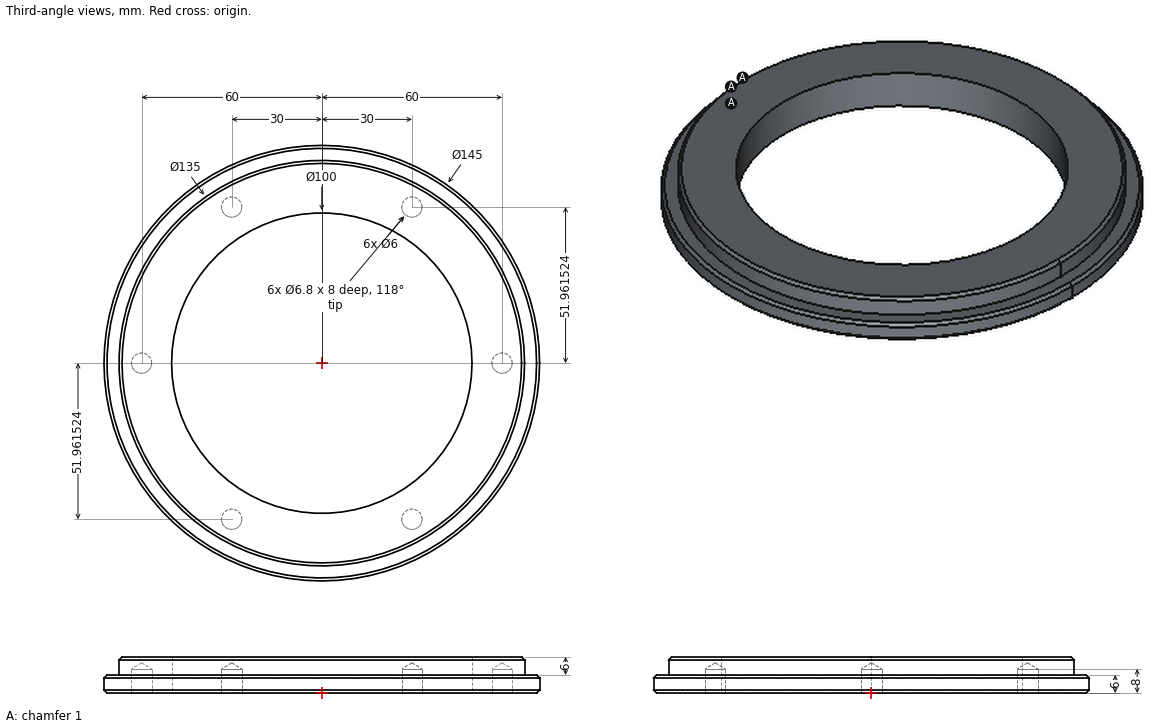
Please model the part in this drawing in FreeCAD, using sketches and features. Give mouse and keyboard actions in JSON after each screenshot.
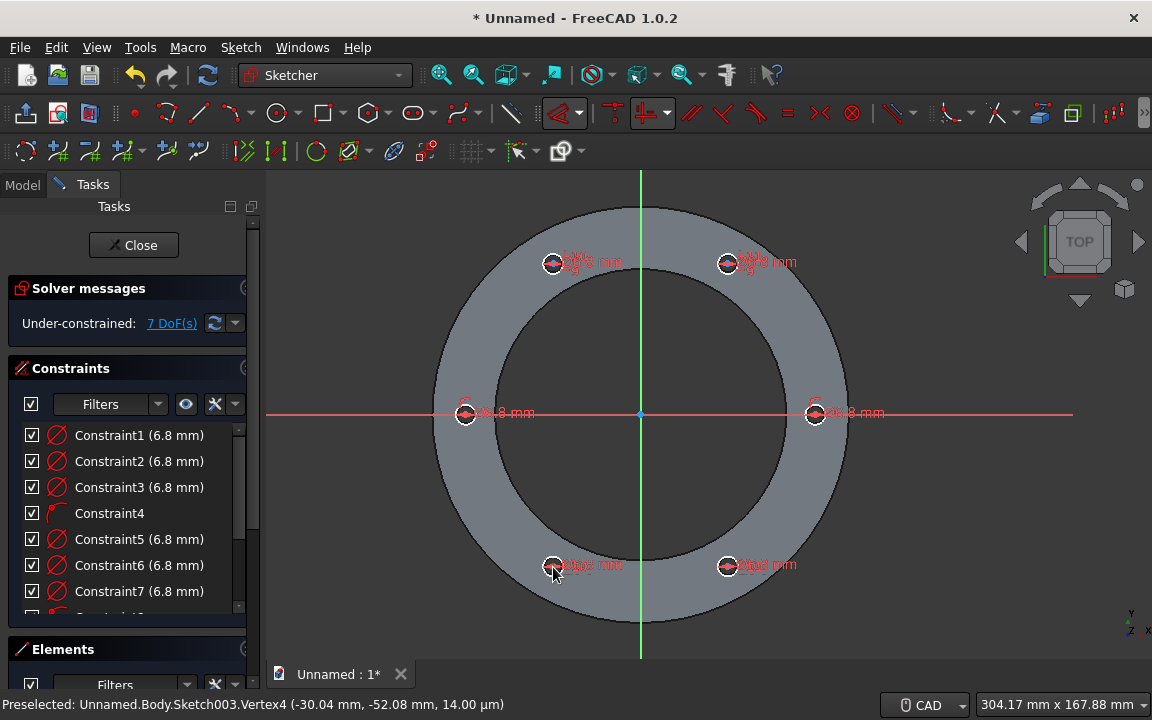
{"action": "left_click", "coordinate": [728, 567]}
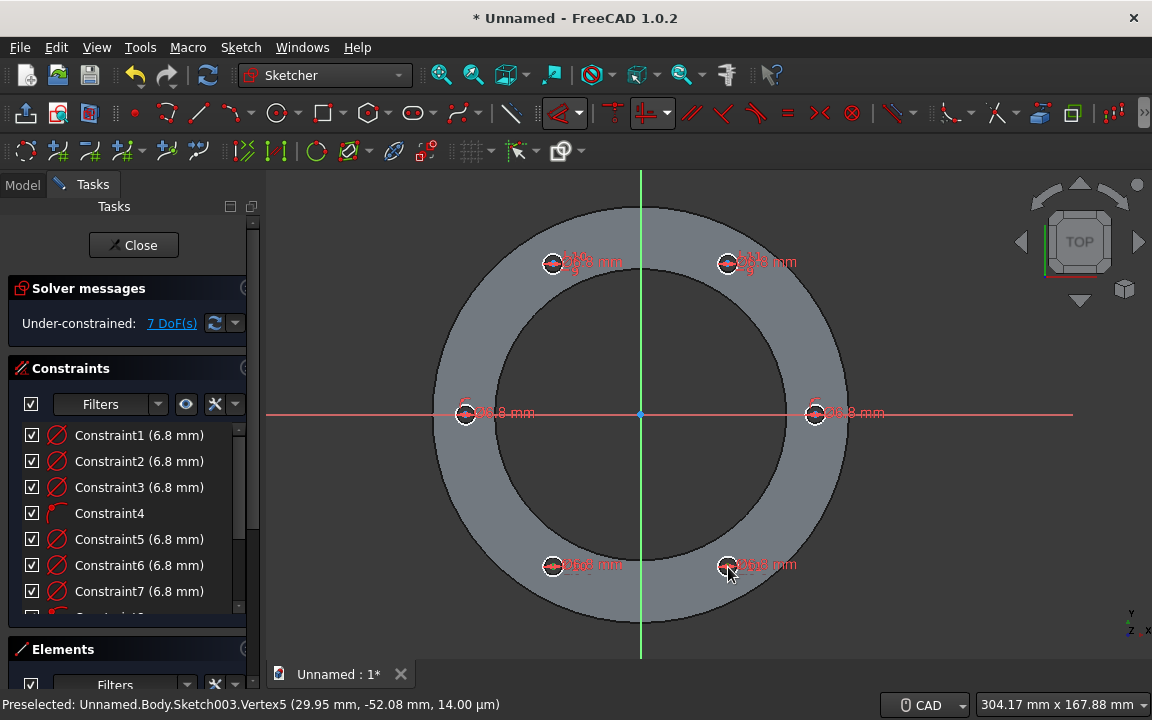
{"action": "left_click", "coordinate": [670, 114]}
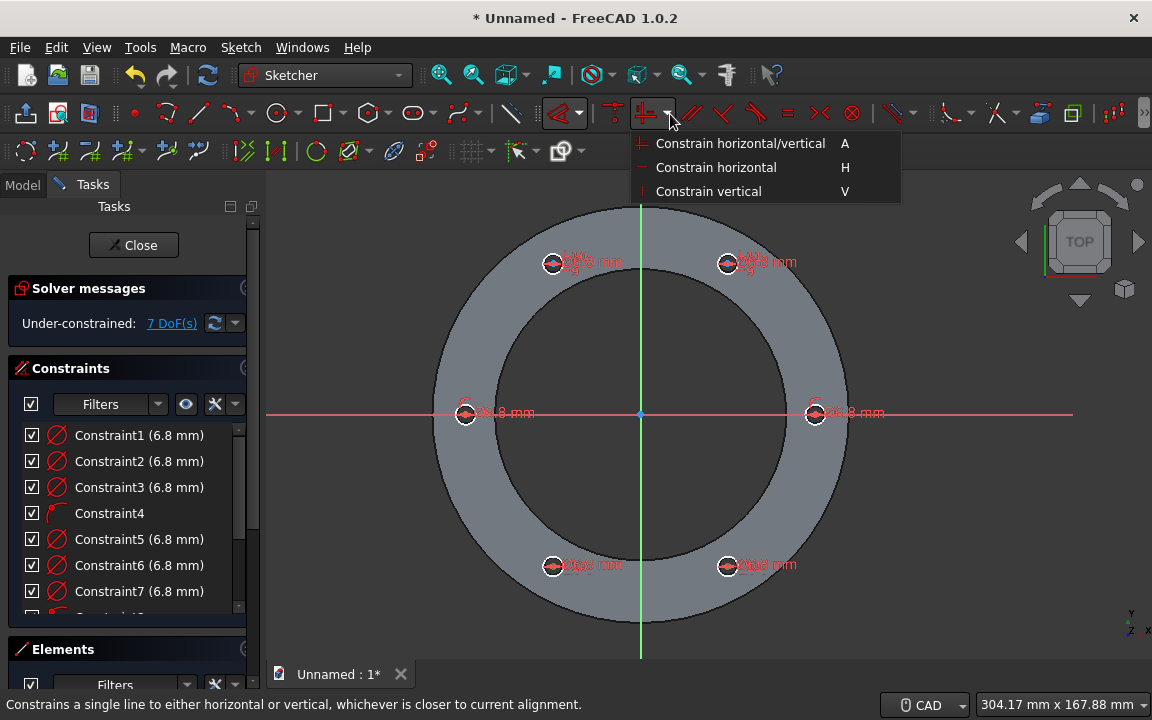
{"action": "left_click", "coordinate": [766, 167]}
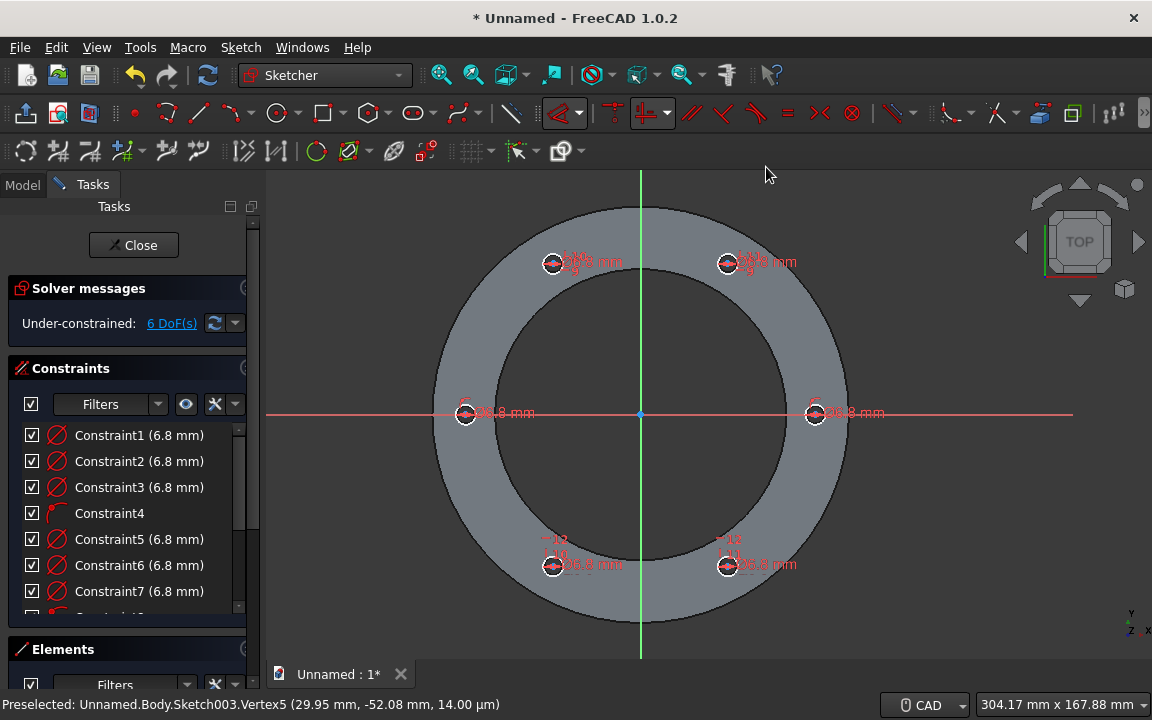
{"action": "left_click", "coordinate": [728, 264]}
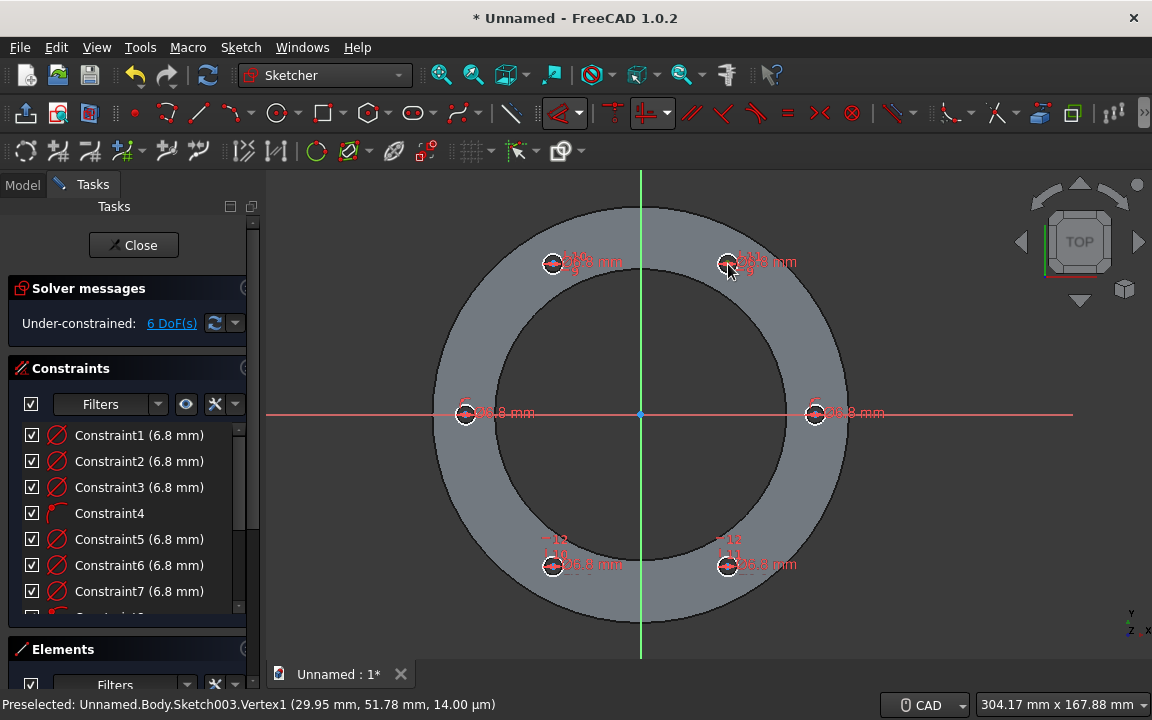
{"action": "key", "text": "l"}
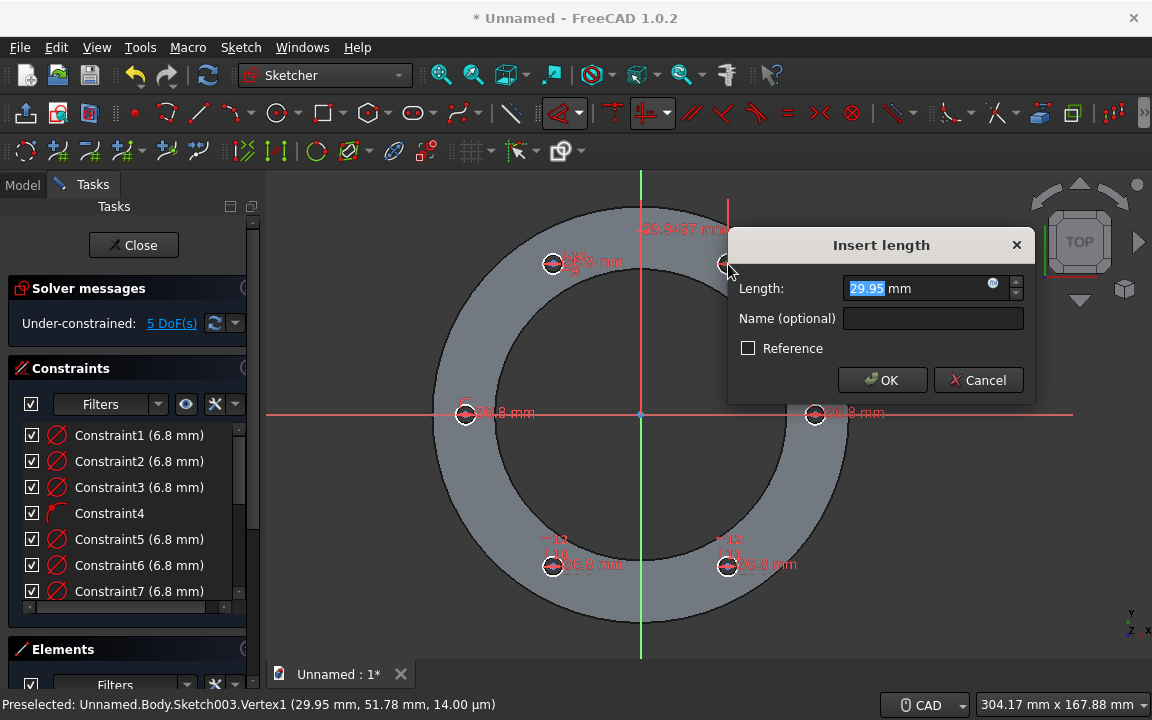
{"action": "type", "text": "30"}
{"action": "key", "text": "Return"}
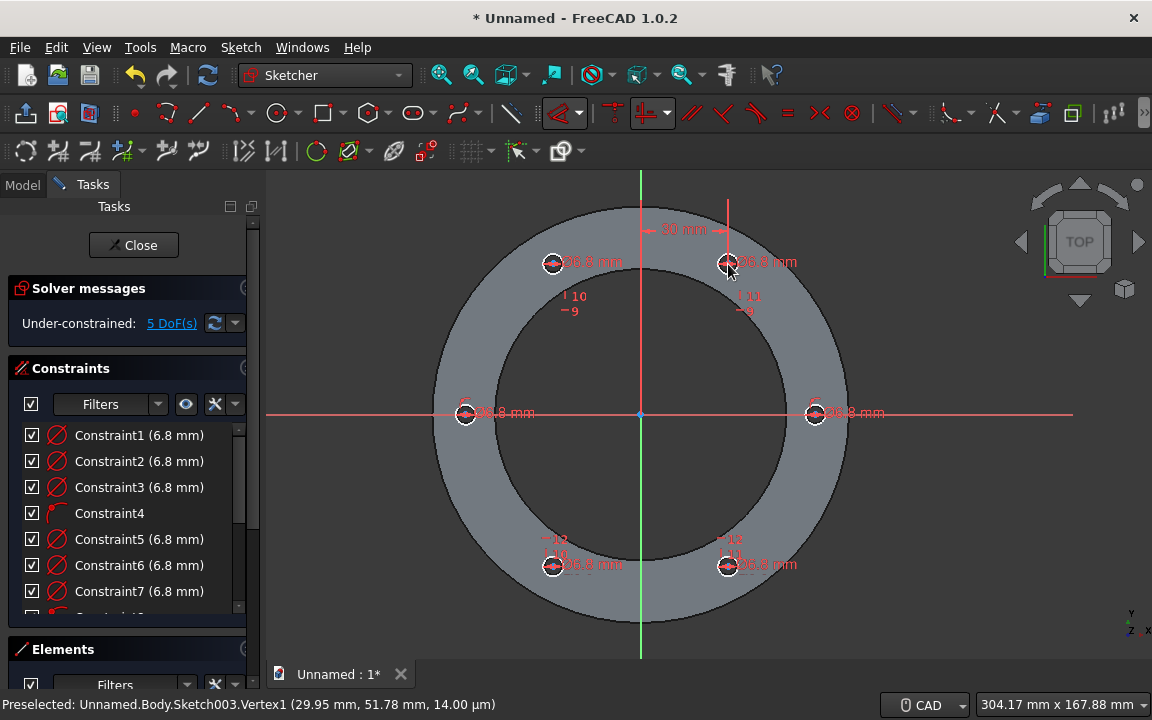
{"action": "left_click", "coordinate": [553, 264]}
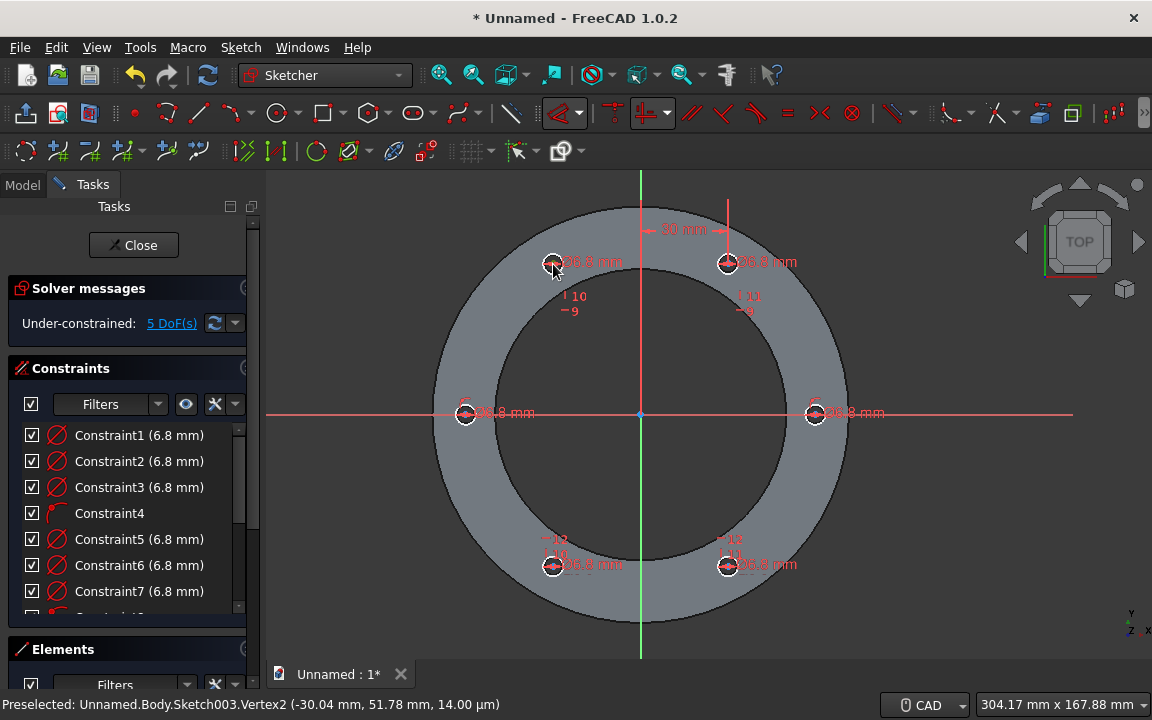
{"action": "left_click", "coordinate": [582, 114]}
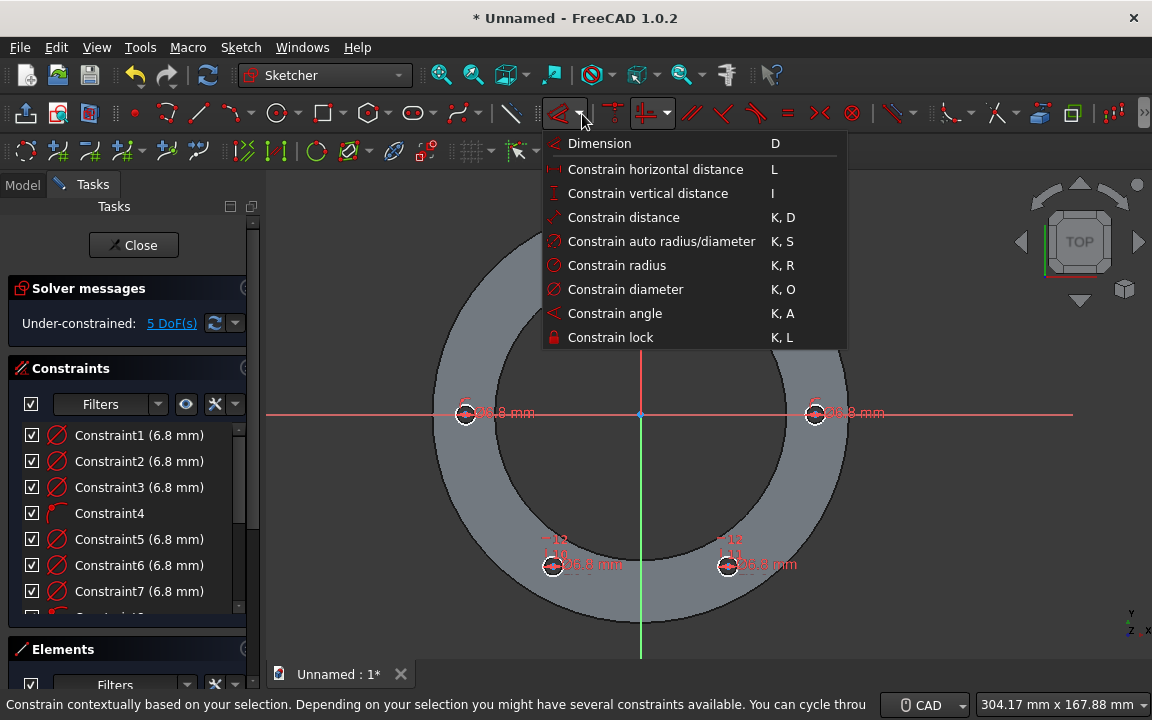
{"action": "left_click", "coordinate": [695, 169]}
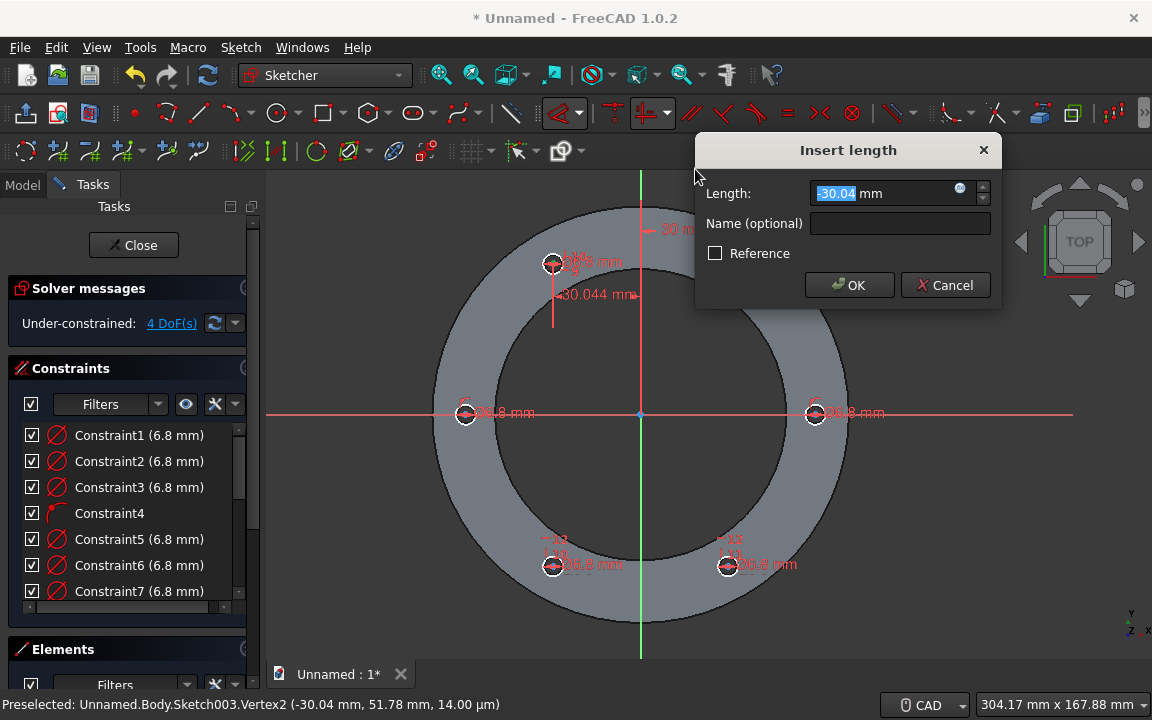
{"action": "type", "text": "-30"}
{"action": "key", "text": "Return"}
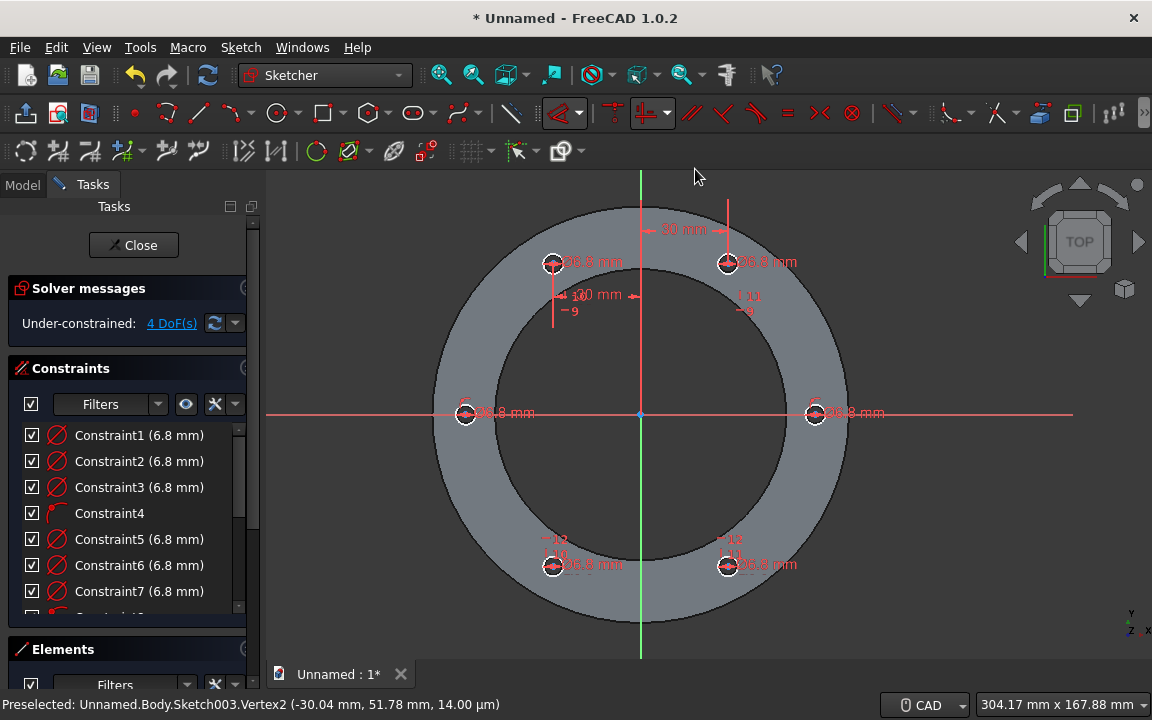
{"action": "left_click", "coordinate": [466, 415]}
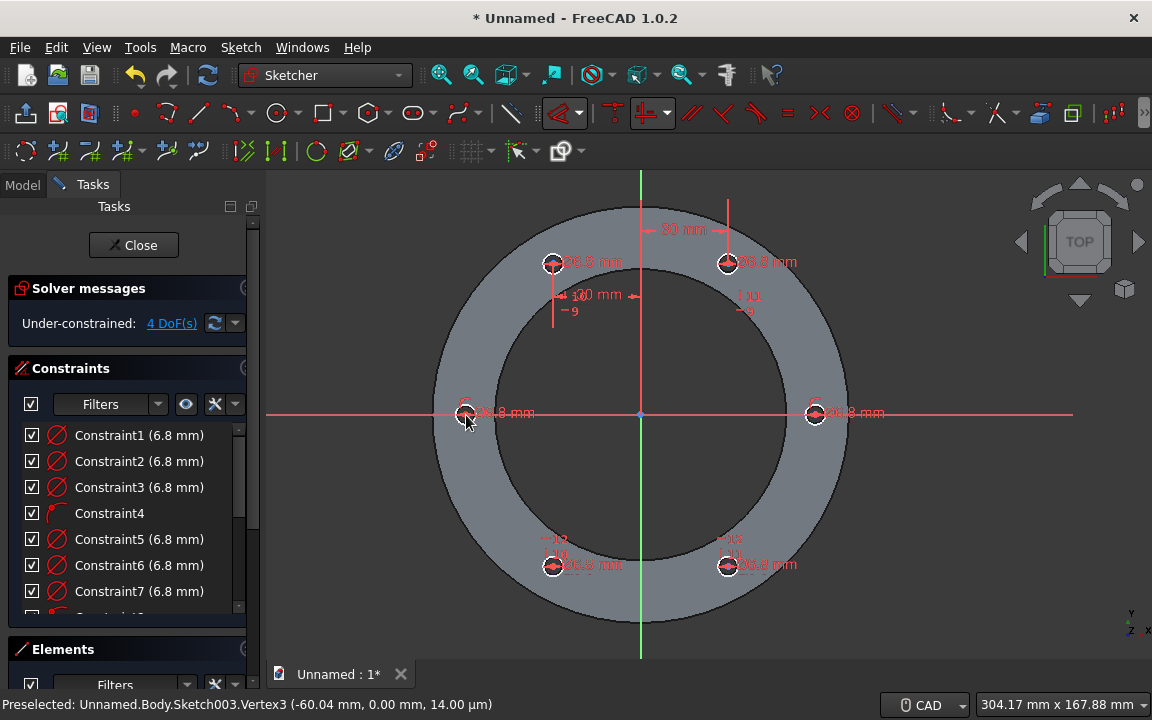
{"action": "left_click", "coordinate": [582, 114]}